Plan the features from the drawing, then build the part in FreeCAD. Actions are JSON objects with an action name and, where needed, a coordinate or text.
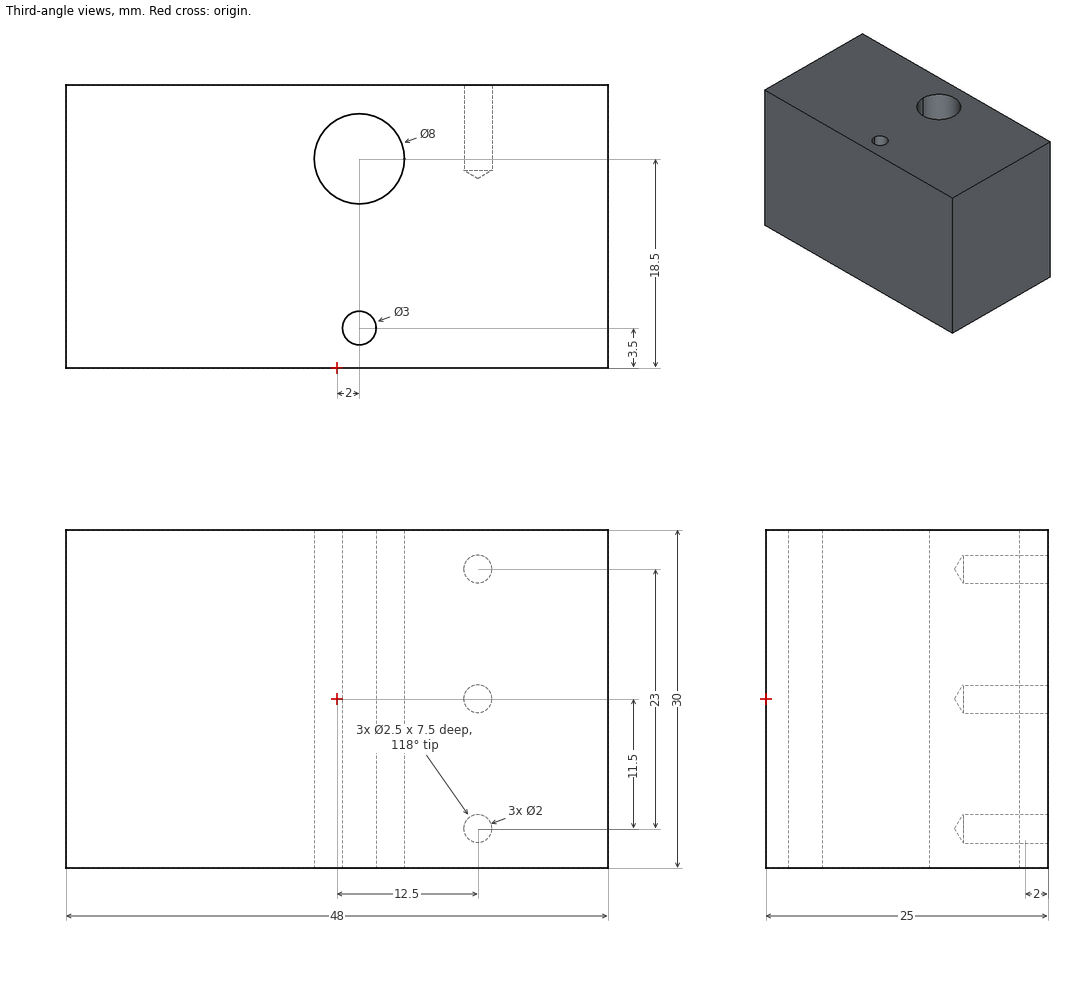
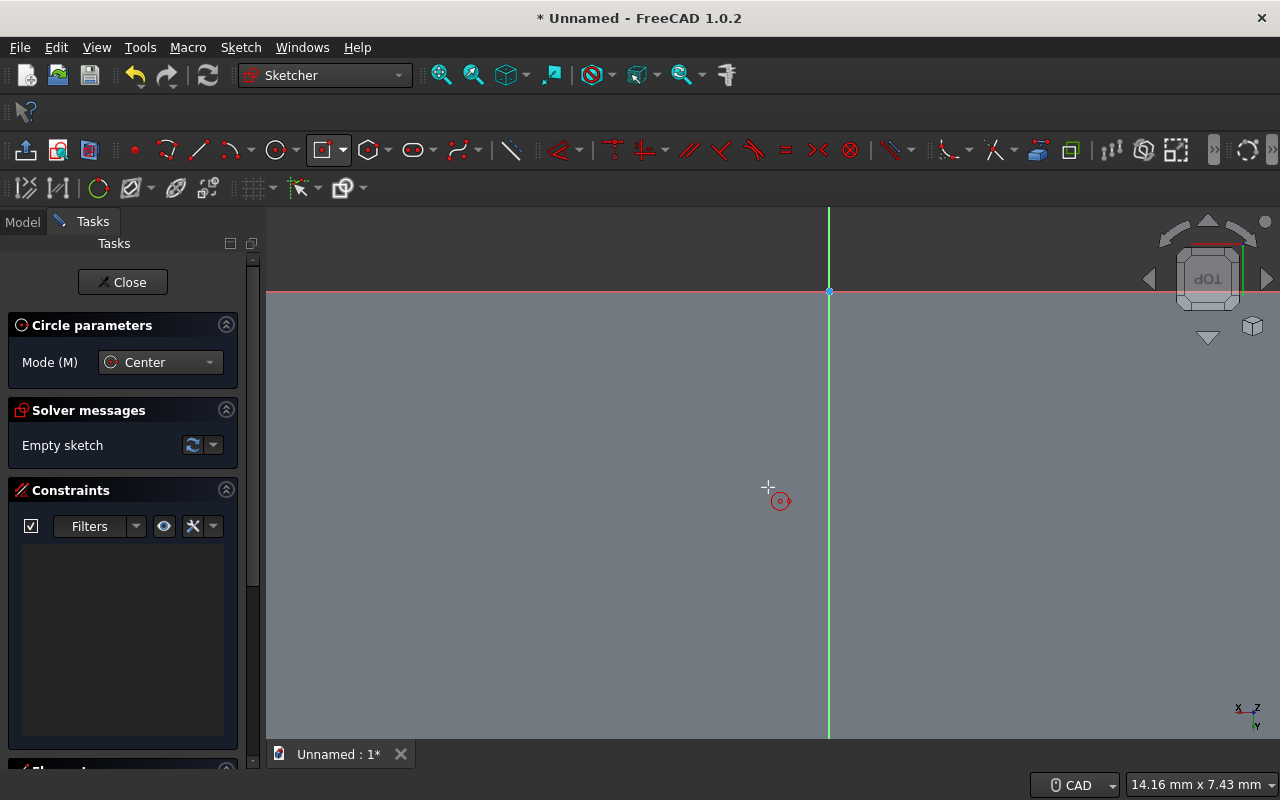
{"action": "left_click", "coordinate": [686, 543]}
{"action": "left_click", "coordinate": [762, 467]}
{"action": "key", "text": "Escape"}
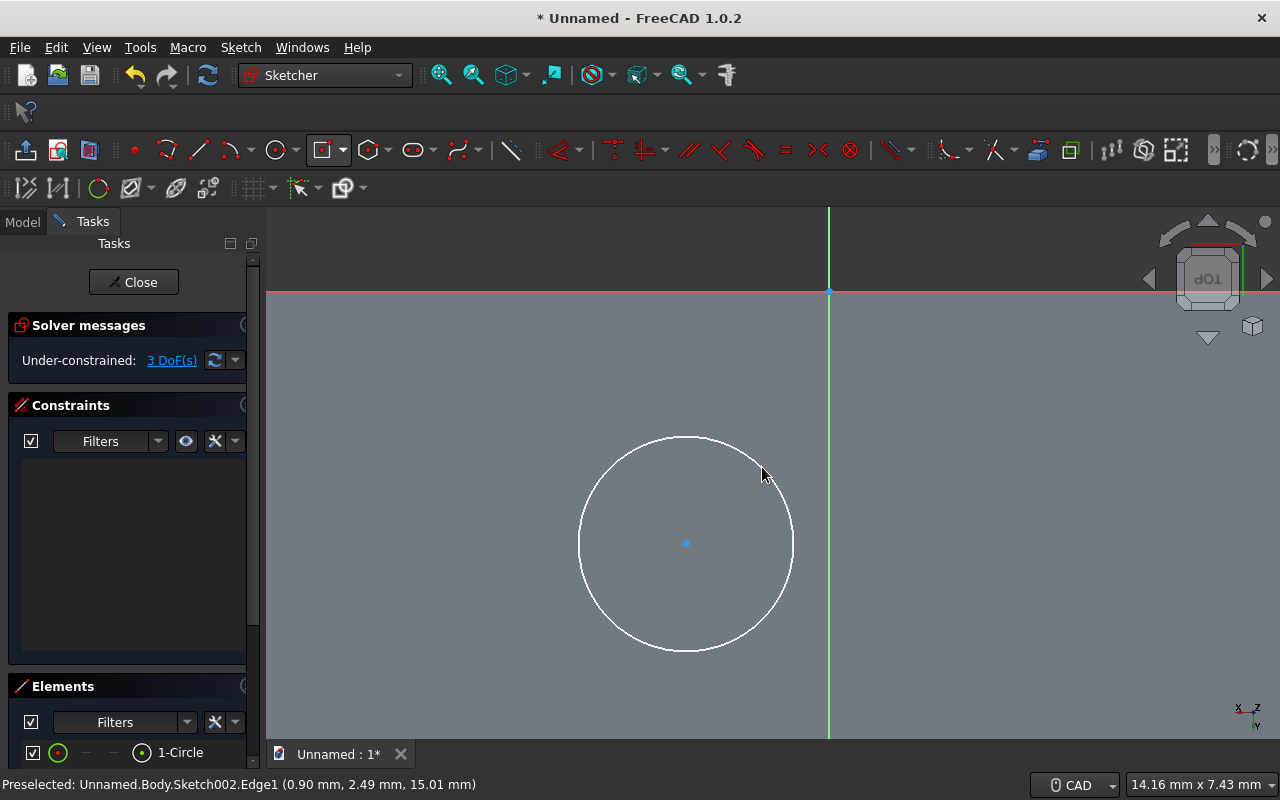
{"action": "key", "text": "d"}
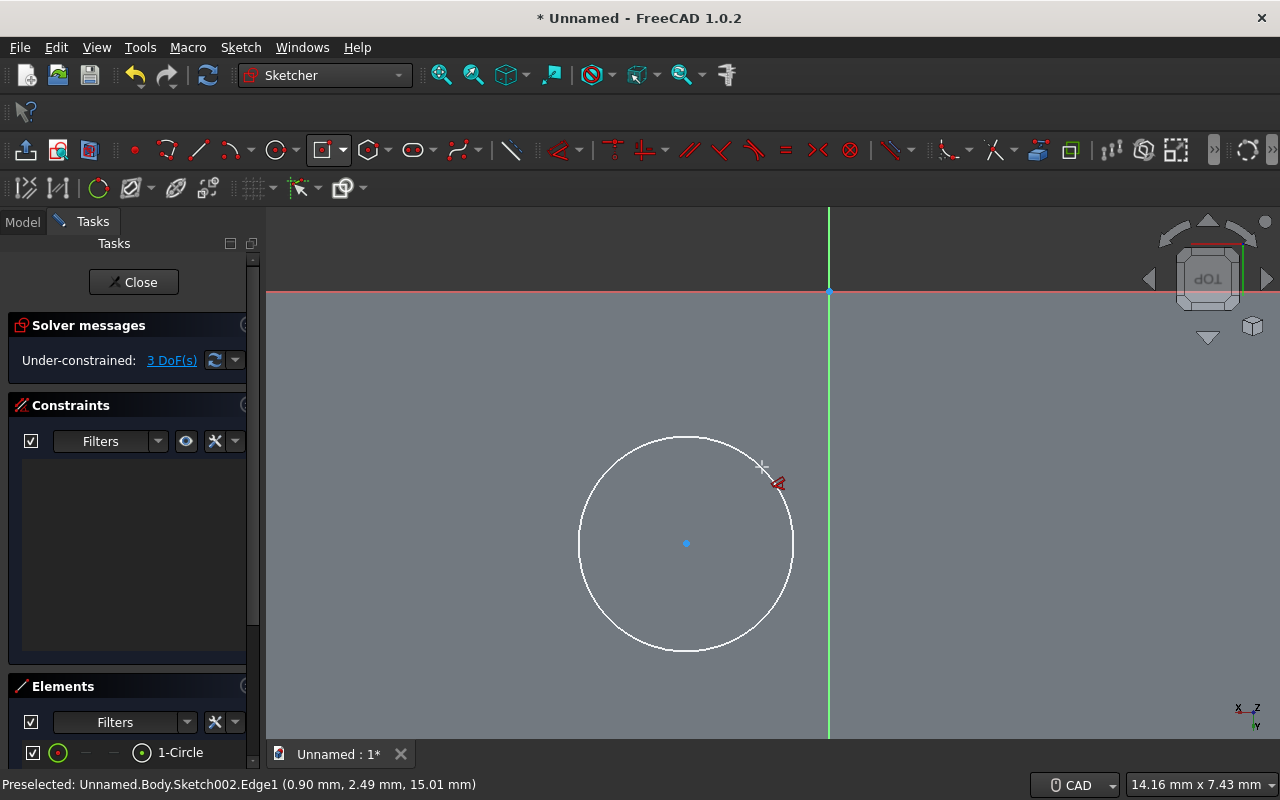
{"action": "left_click", "coordinate": [762, 468]}
{"action": "left_click", "coordinate": [785, 445]}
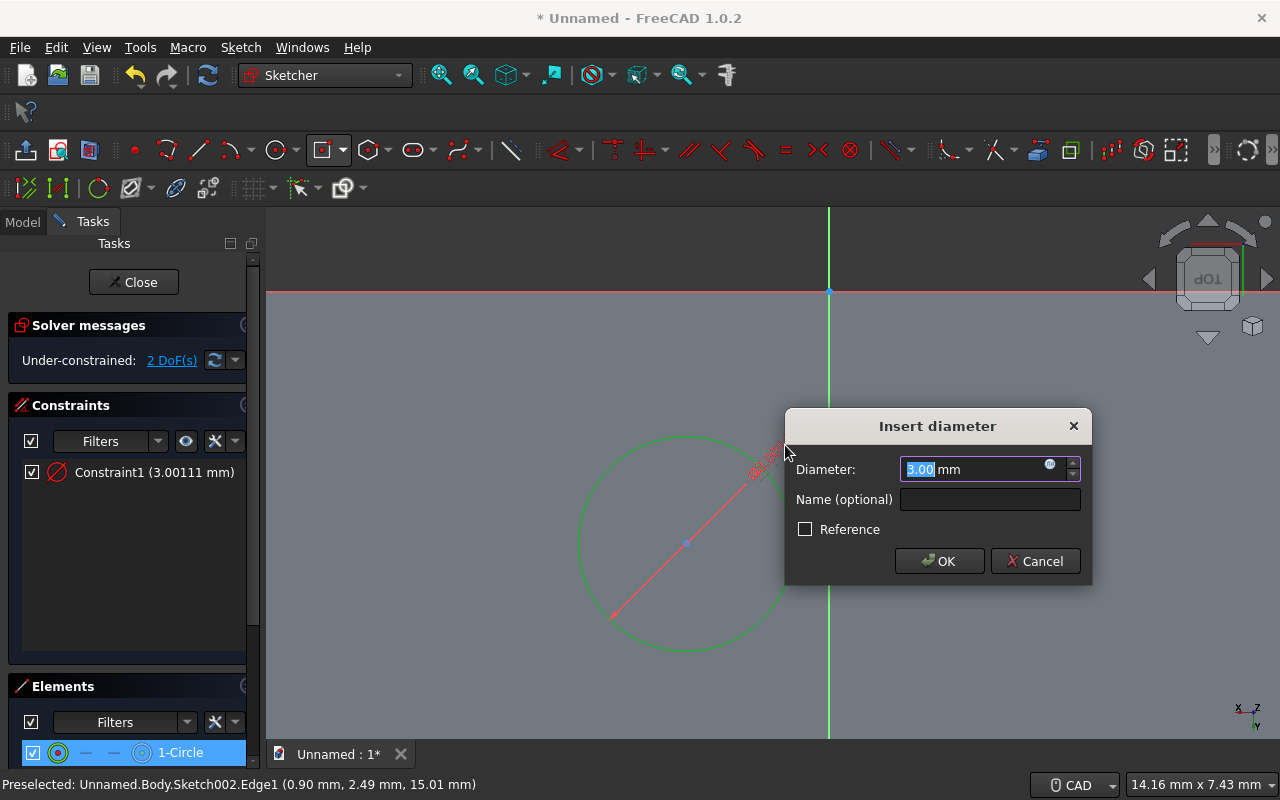
{"action": "type", "text": "3"}
{"action": "key", "text": "Return"}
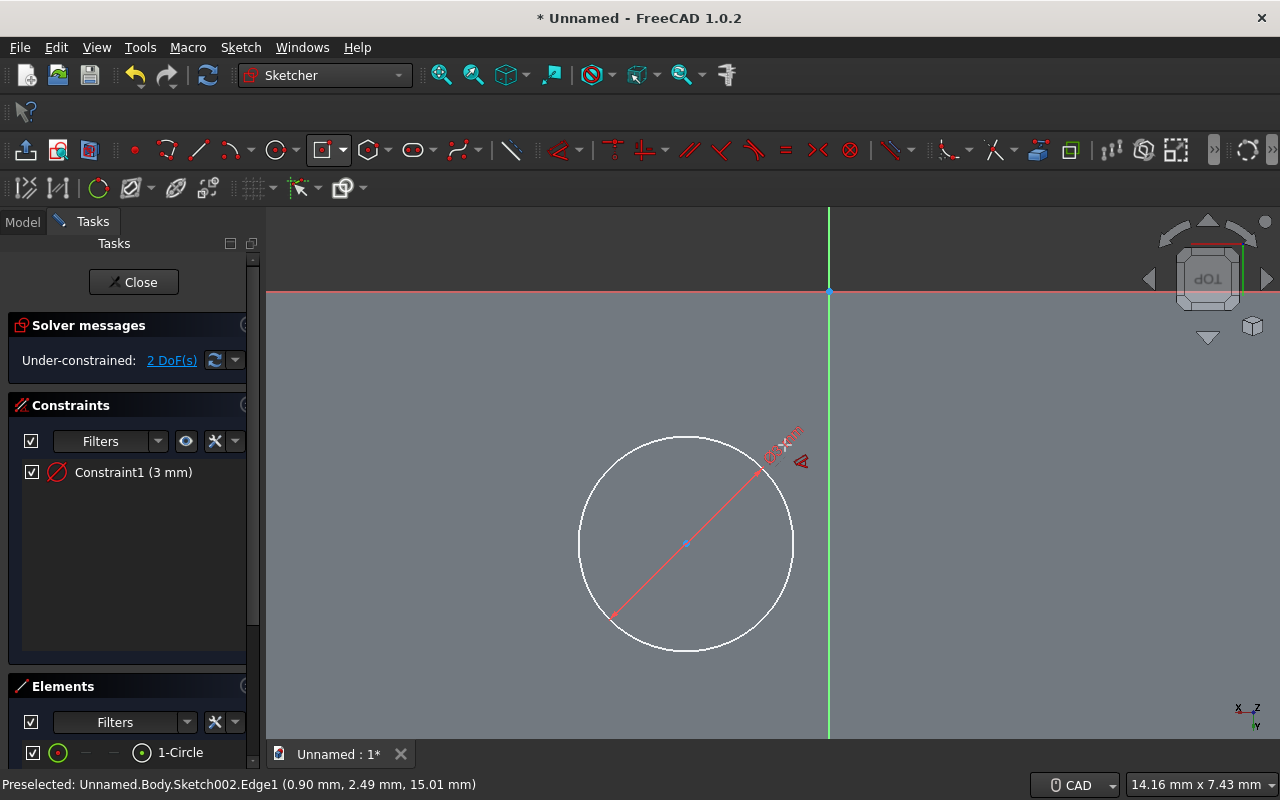
{"action": "left_click", "coordinate": [686, 544]}
{"action": "left_click", "coordinate": [758, 258]}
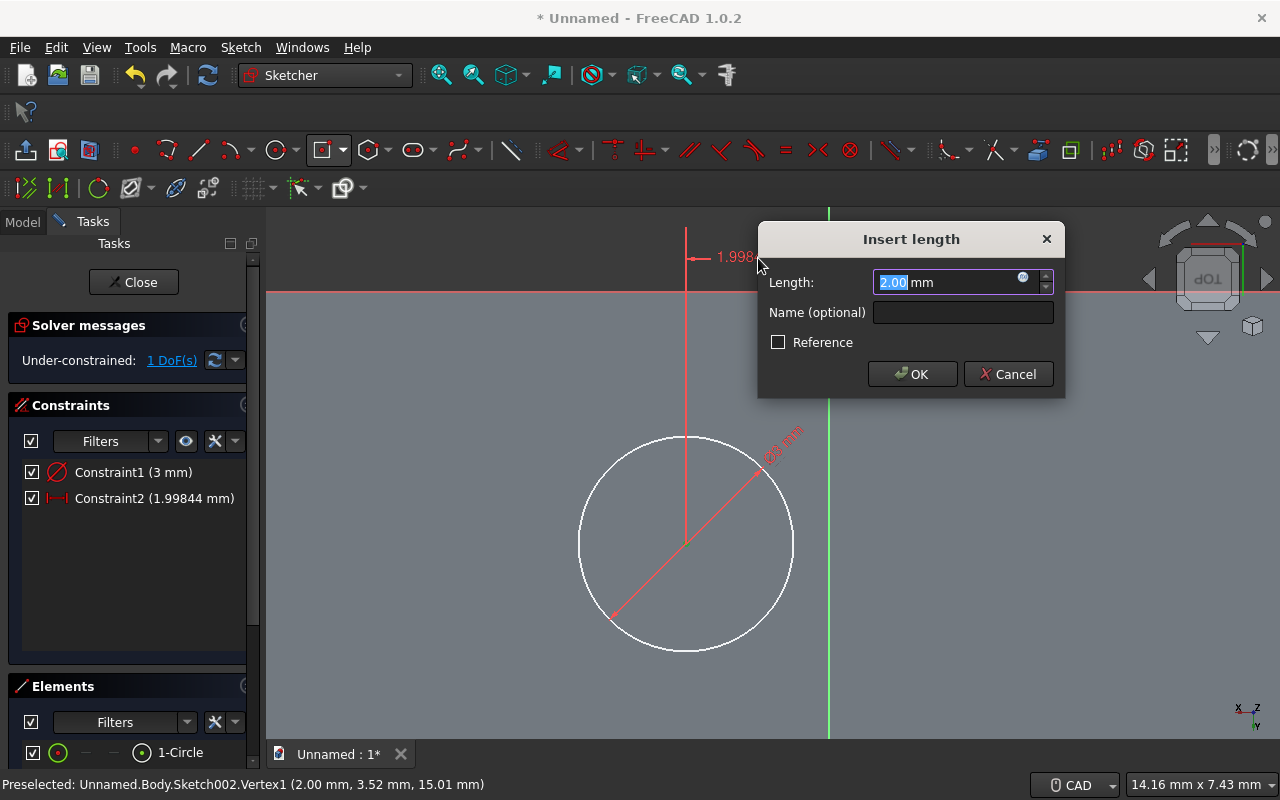
{"action": "type", "text": "2"}
{"action": "key", "text": "Return"}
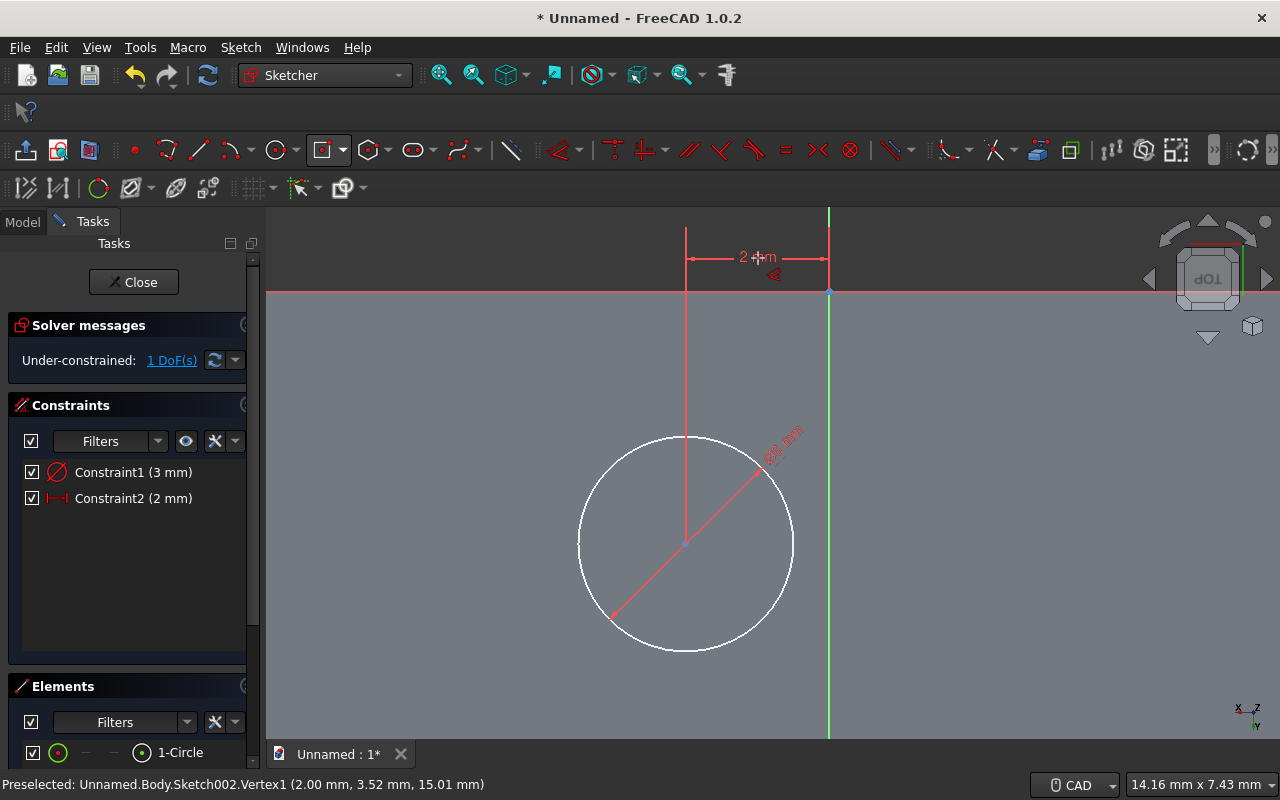
{"action": "left_click", "coordinate": [686, 544]}
{"action": "left_click", "coordinate": [863, 418]}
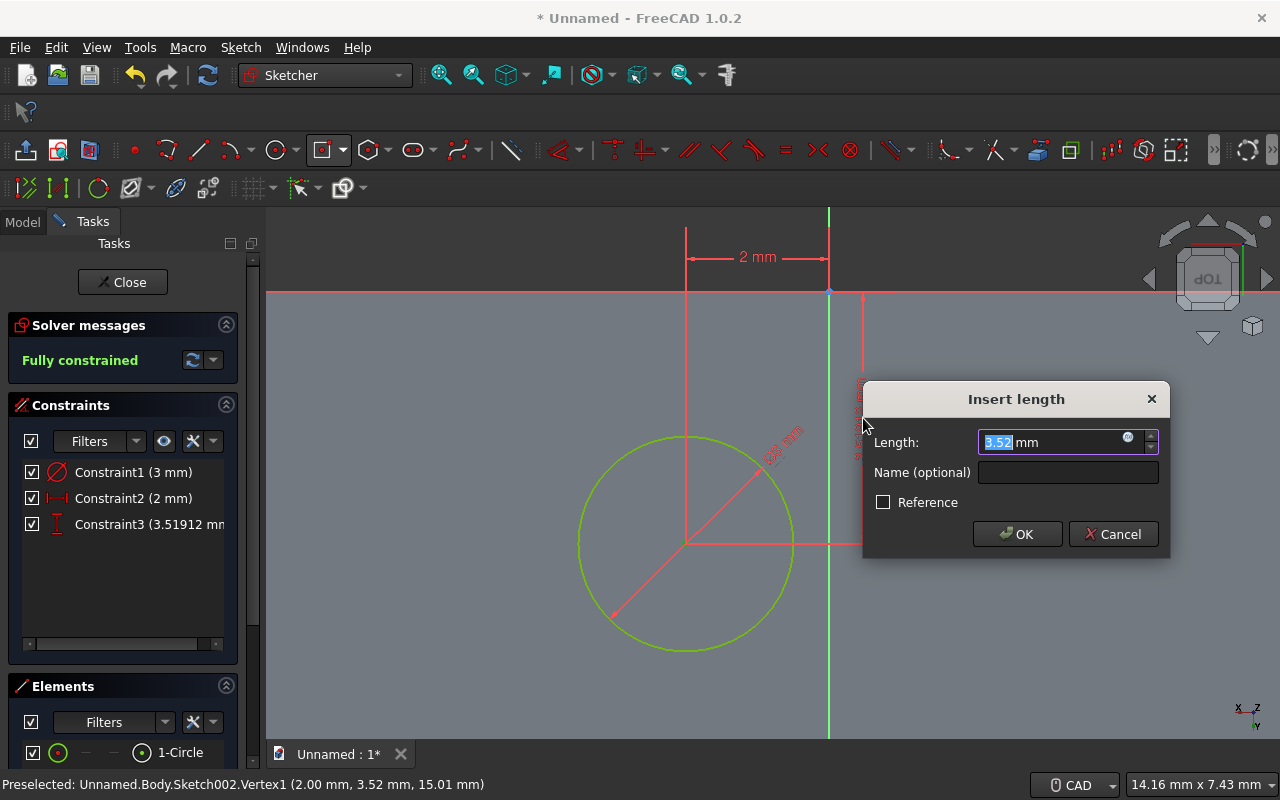
{"action": "type", "text": "3.5"}
{"action": "key", "text": "Return"}
{"action": "key", "text": "Escape"}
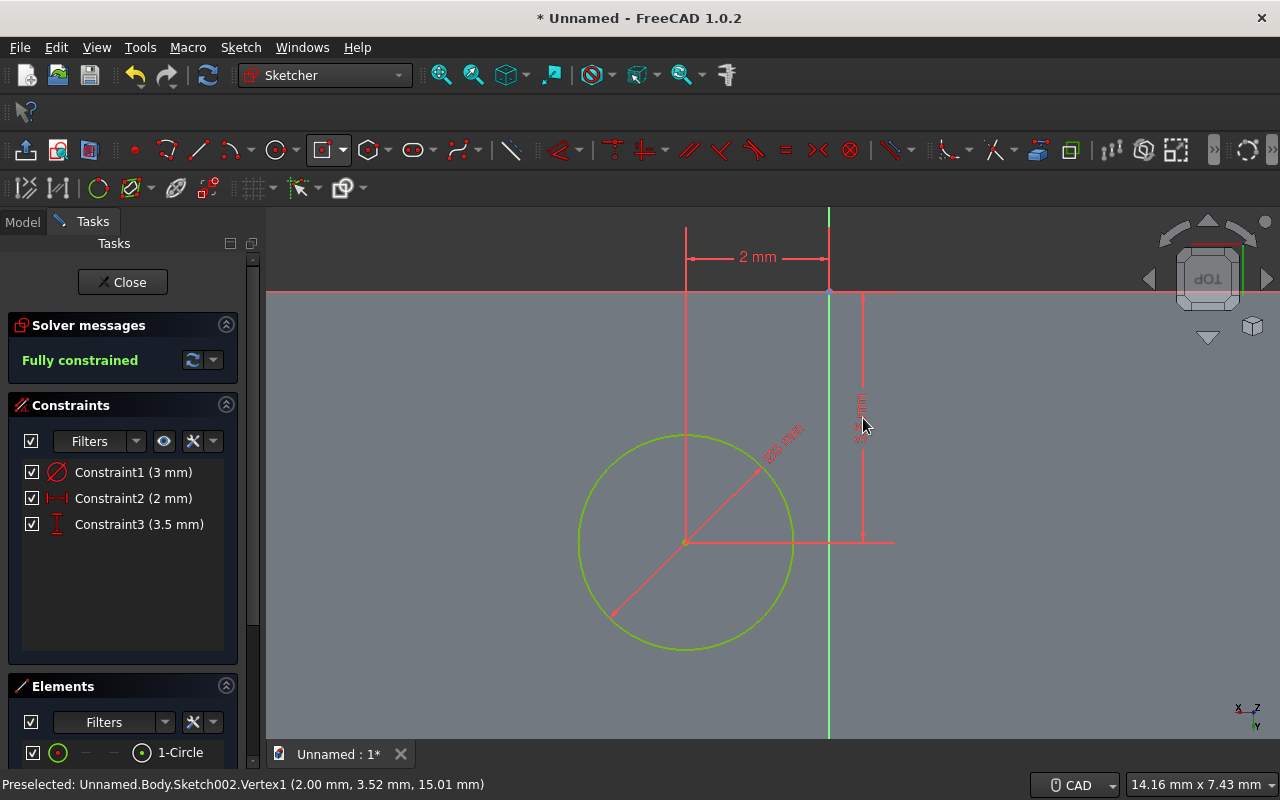
{"action": "left_click", "coordinate": [123, 282]}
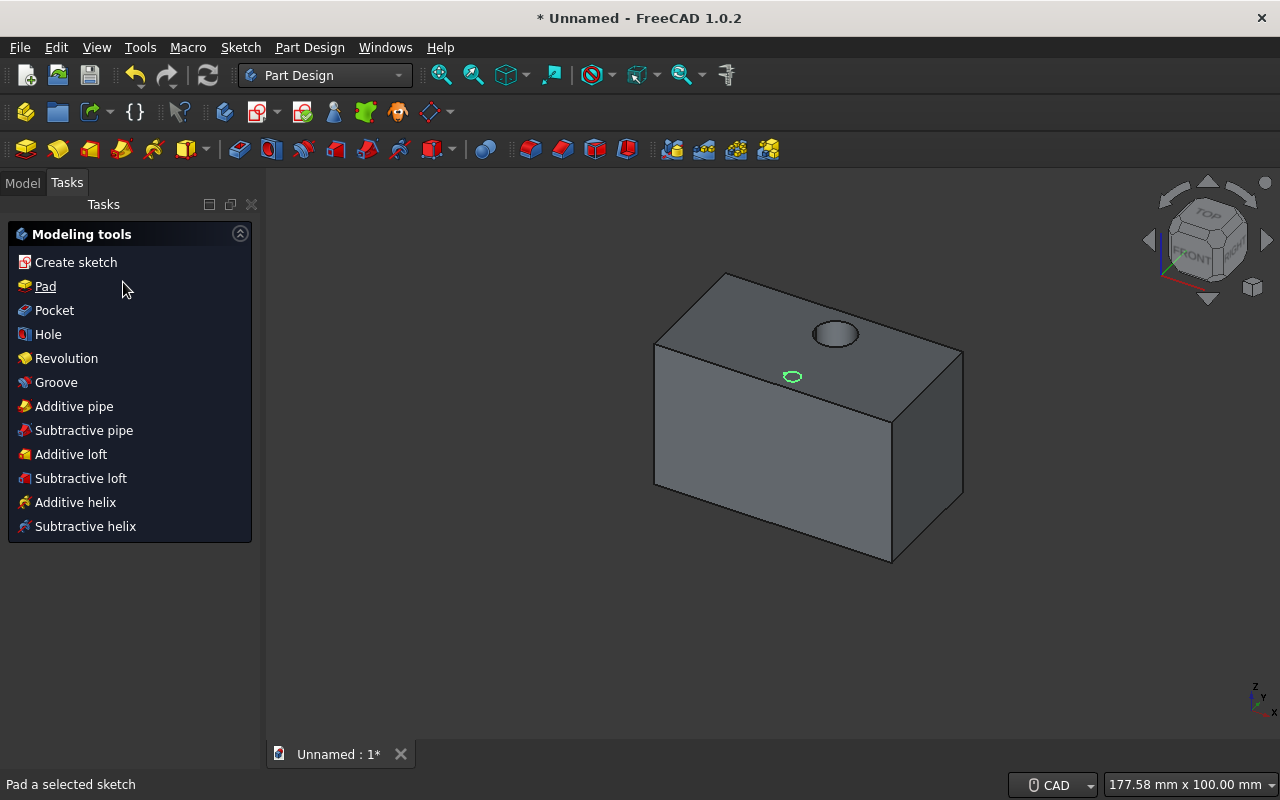
{"action": "left_click", "coordinate": [240, 150]}